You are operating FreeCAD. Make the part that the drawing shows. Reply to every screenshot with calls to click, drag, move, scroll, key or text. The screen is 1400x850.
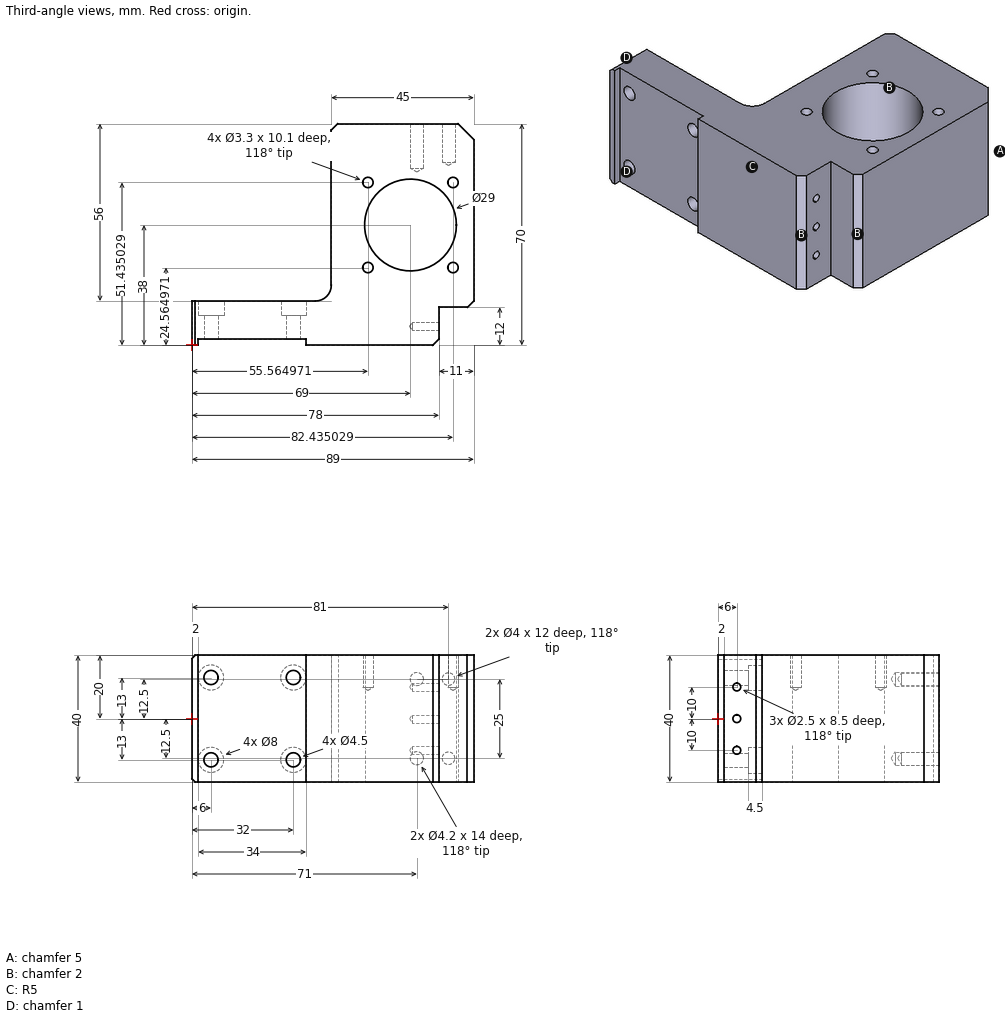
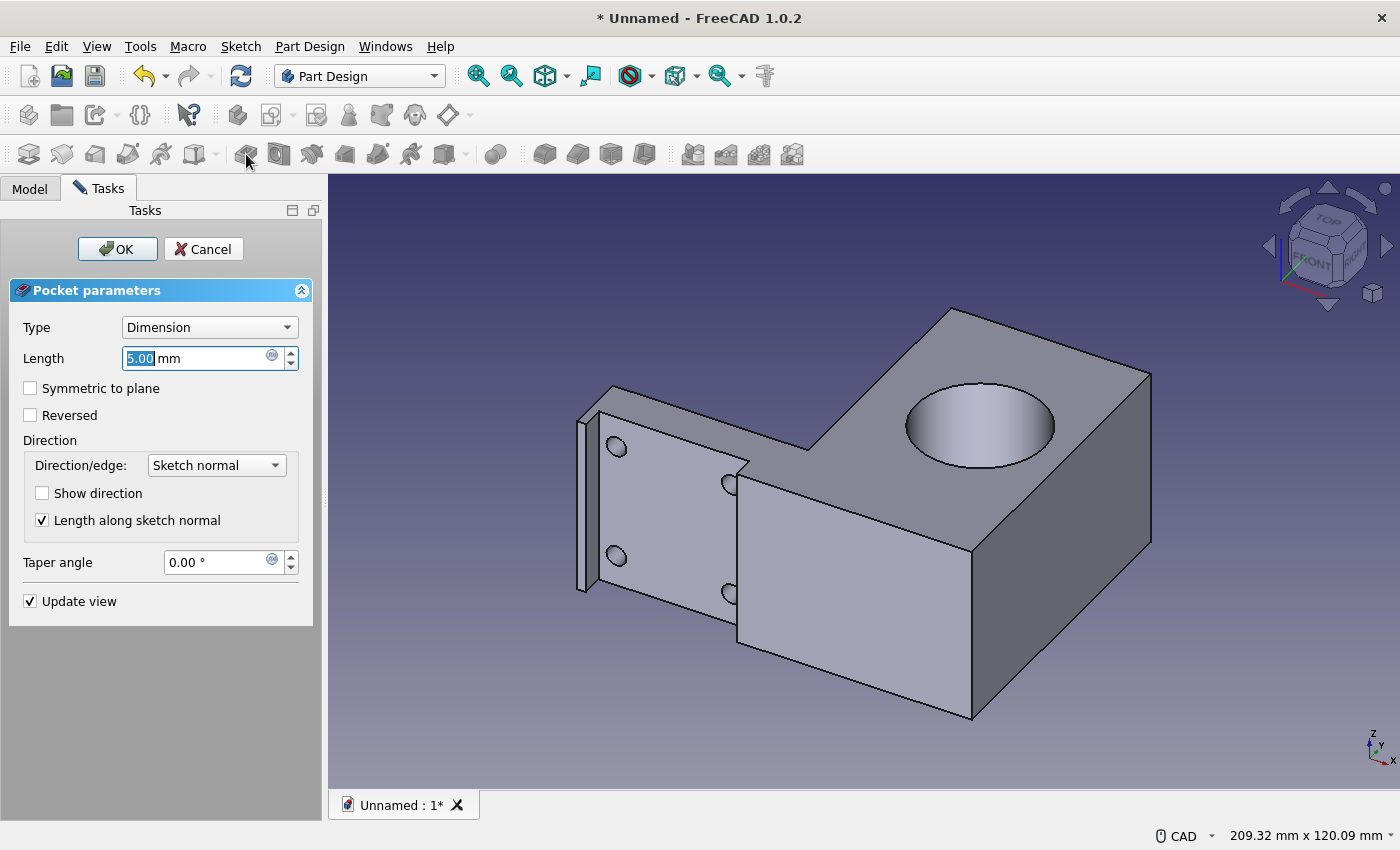
text(2)
key(Tab)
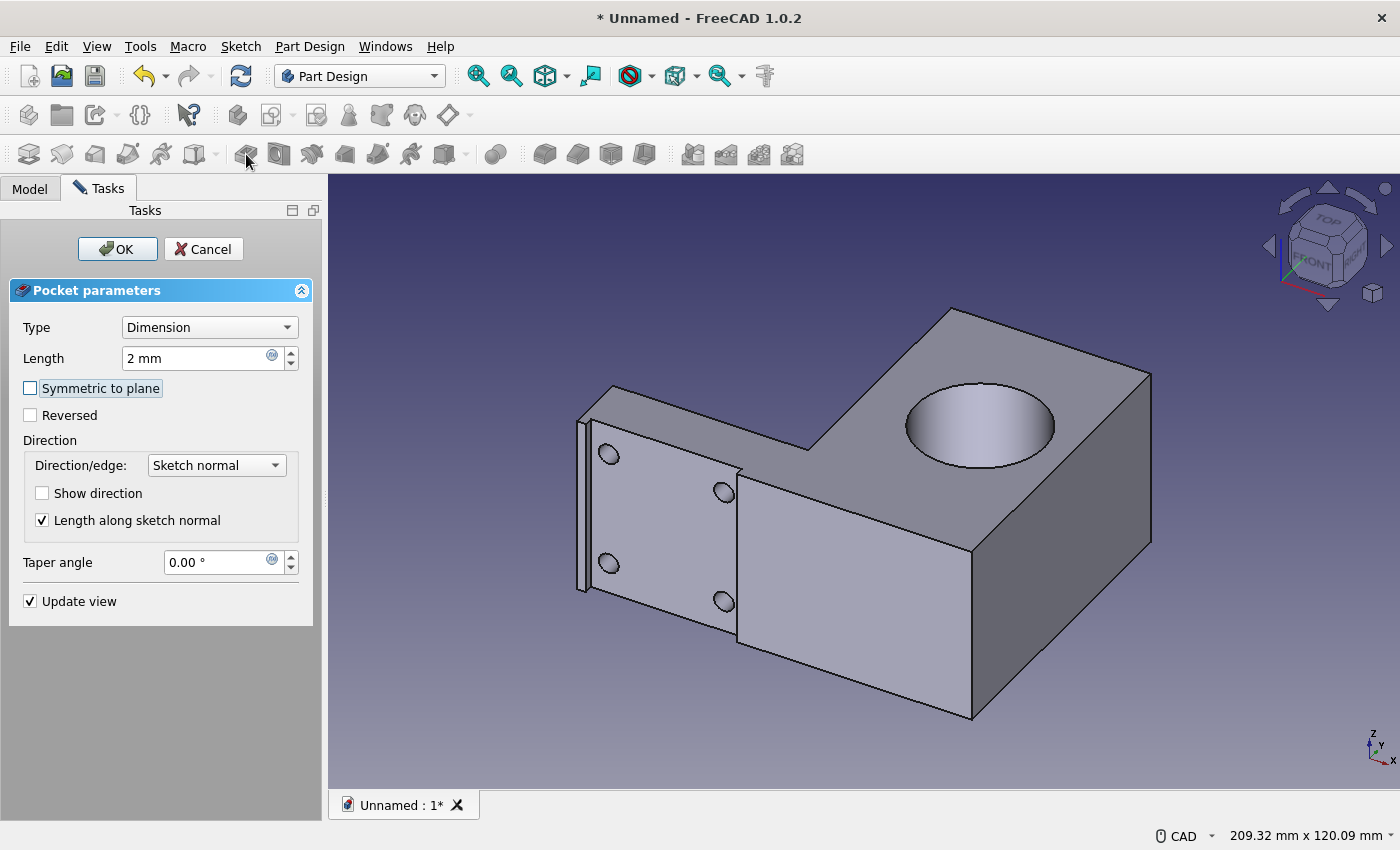
click(118, 249)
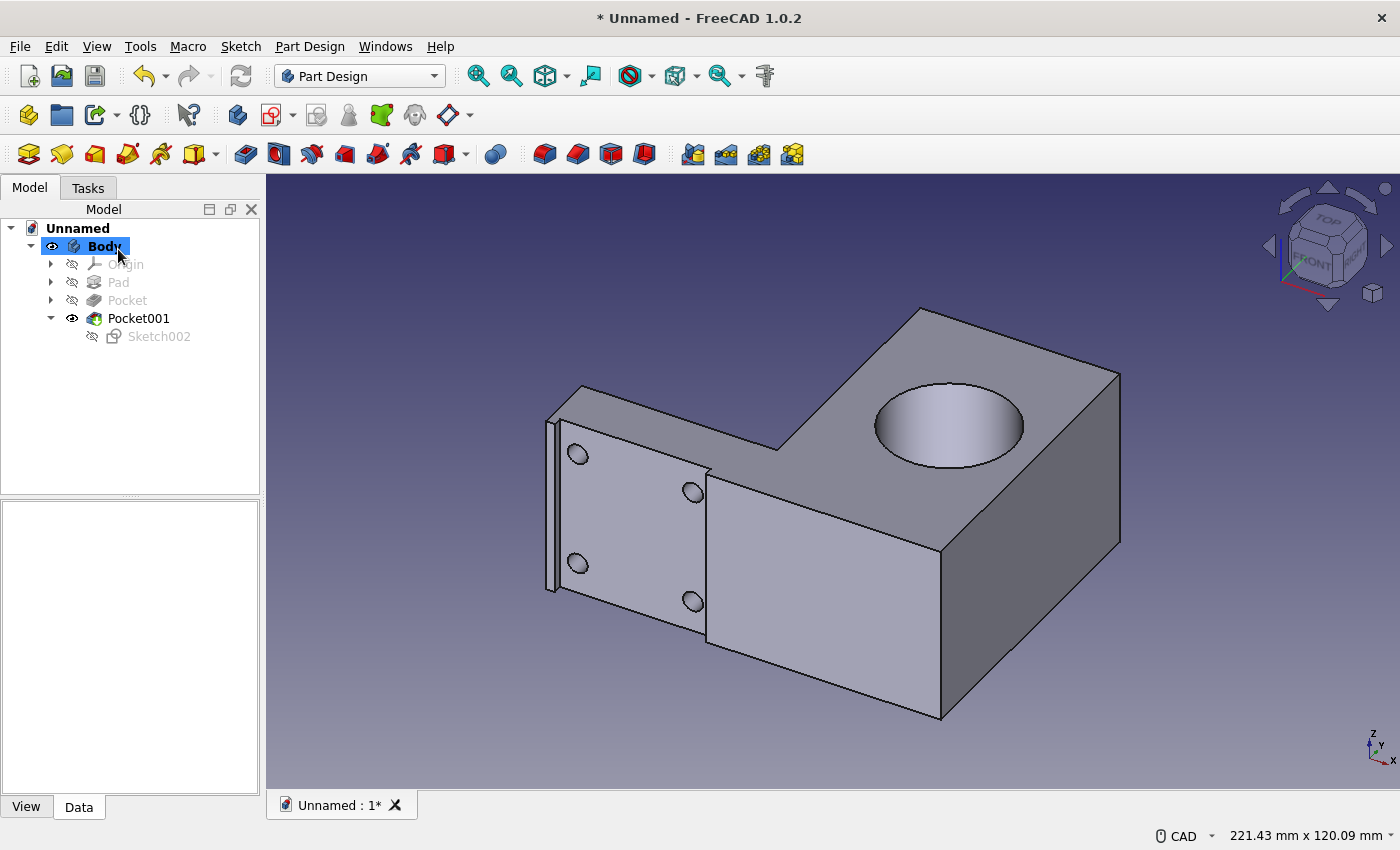
click(838, 466)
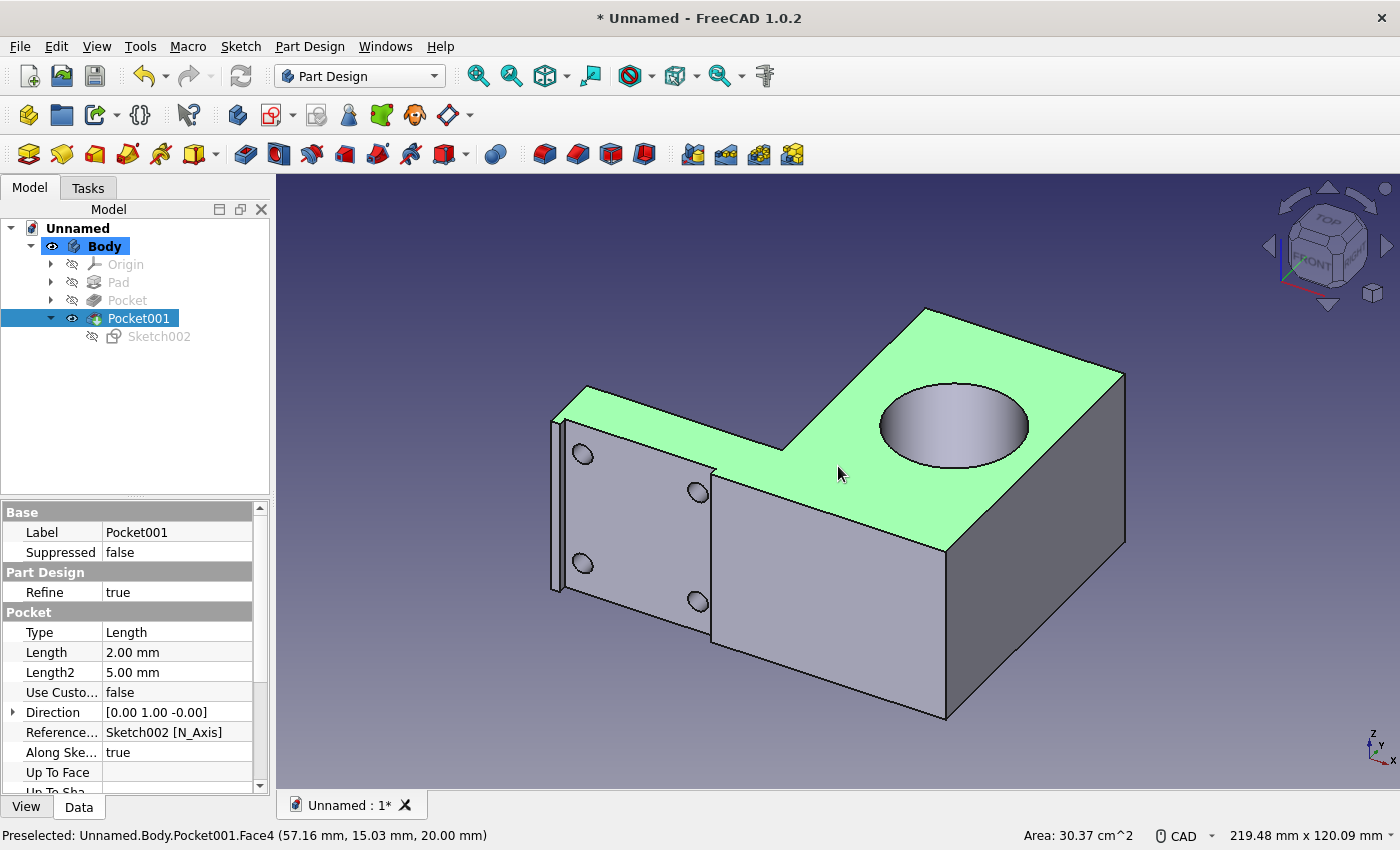
click(270, 116)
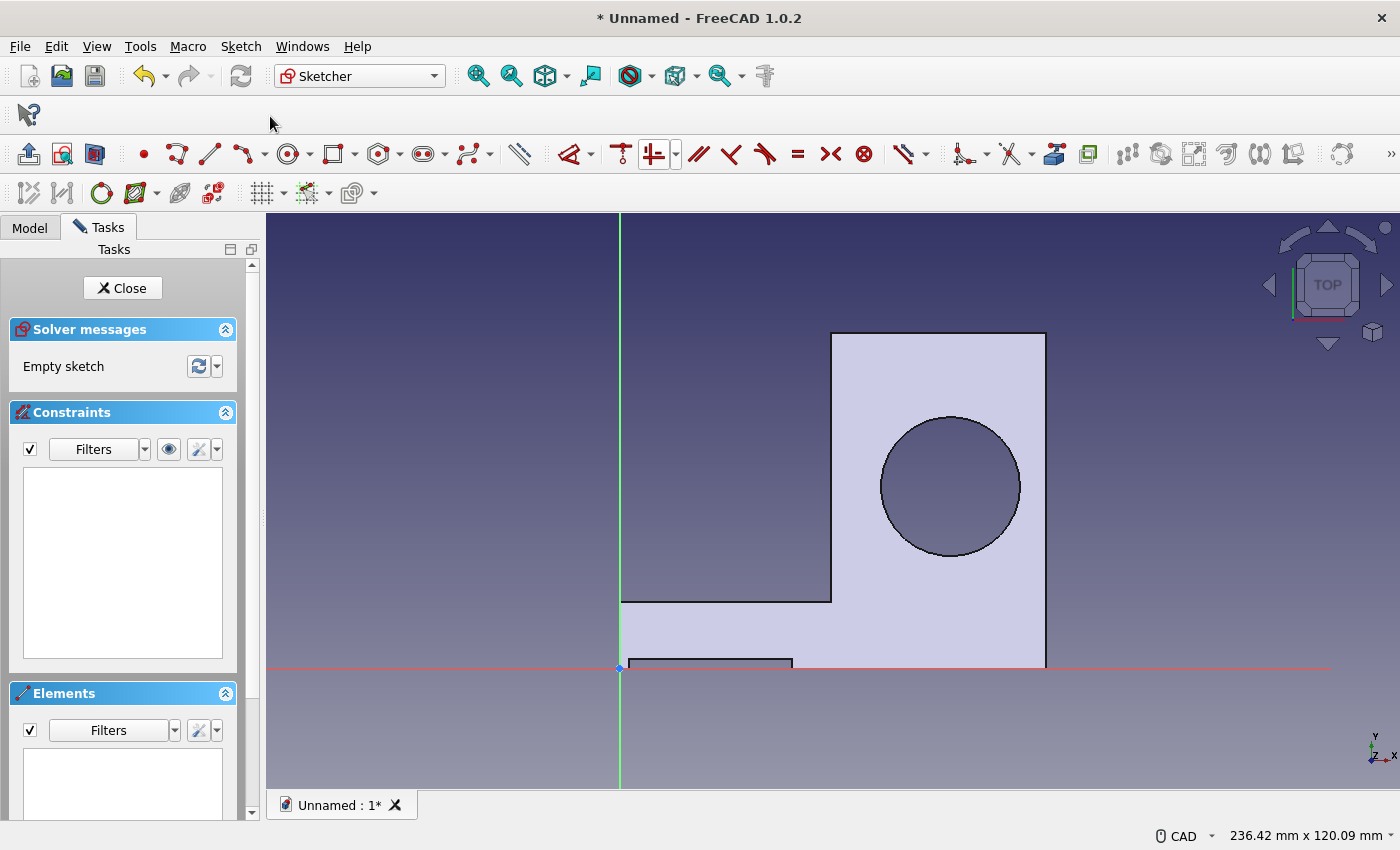
scroll(1059, 478, up, 5)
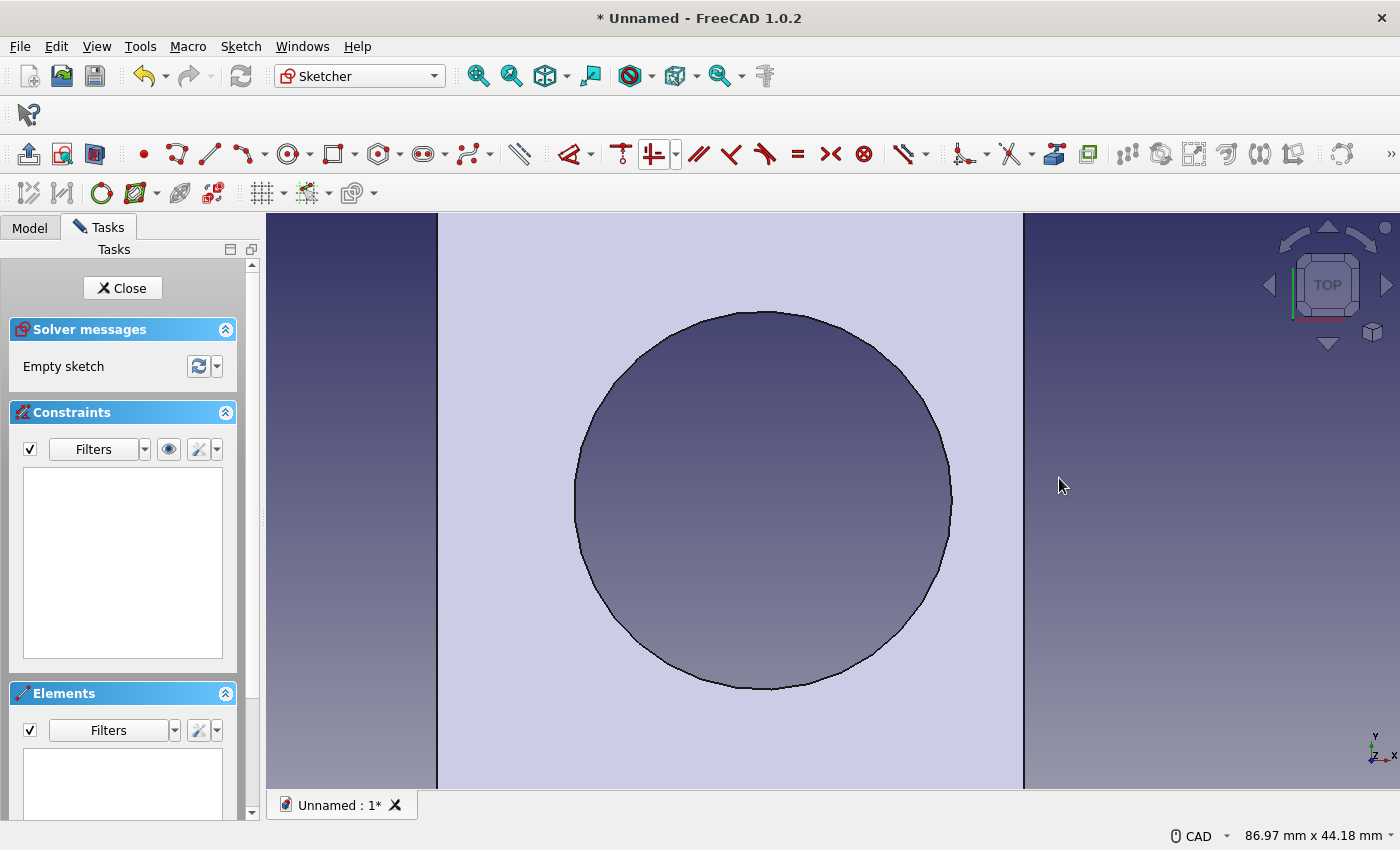
click(288, 154)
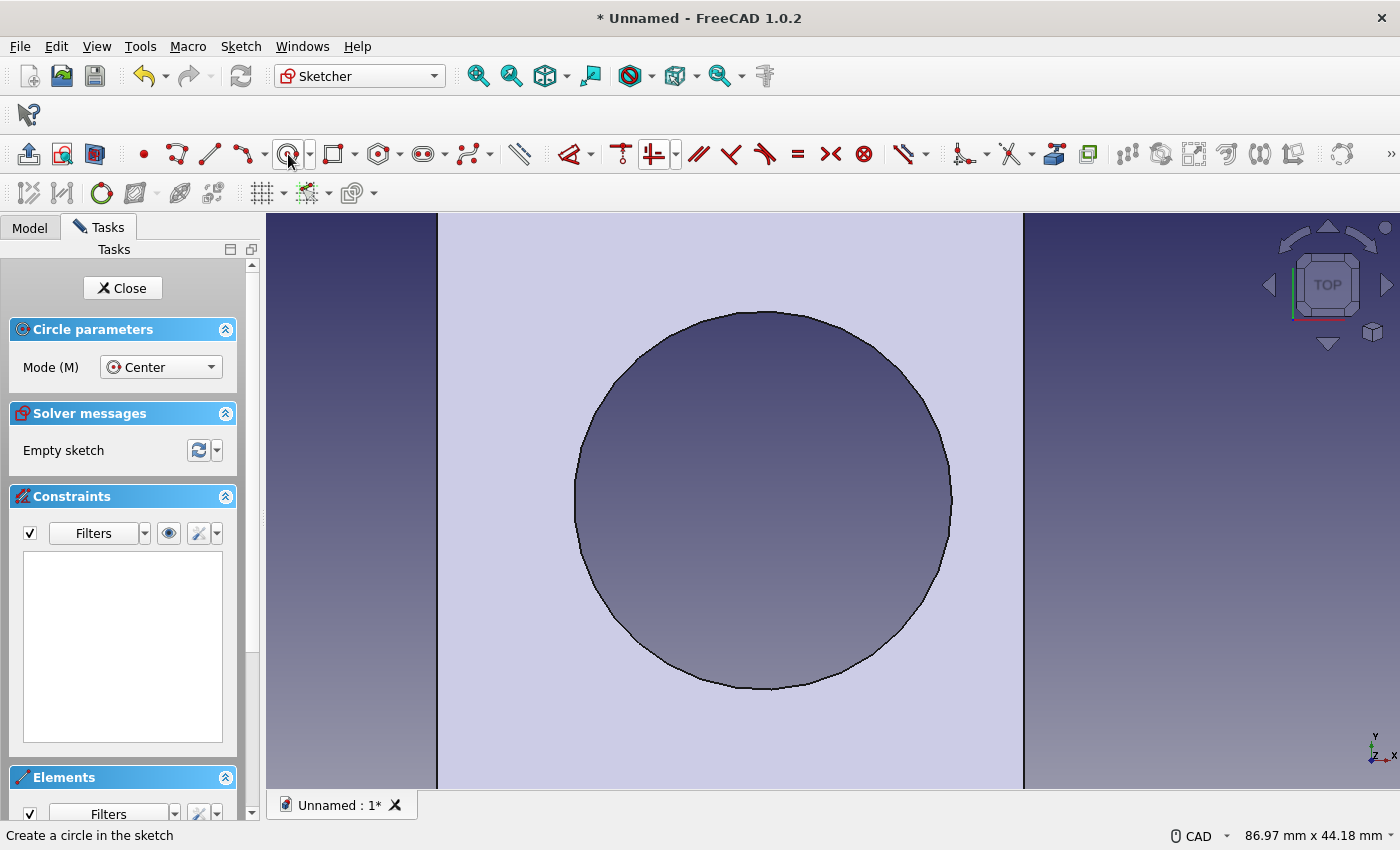
click(588, 325)
move(603, 310)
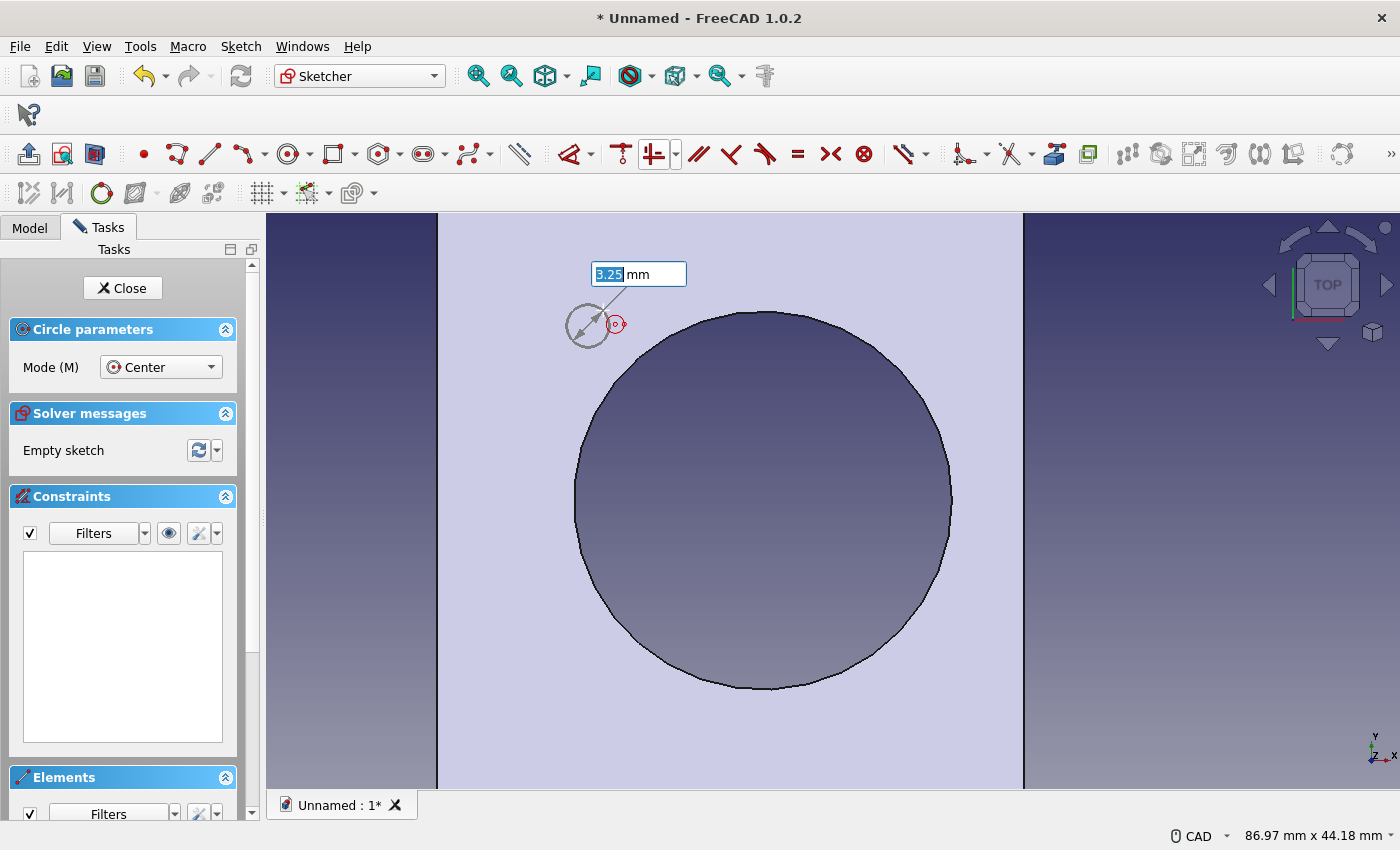
text(3.3)
key(Return)